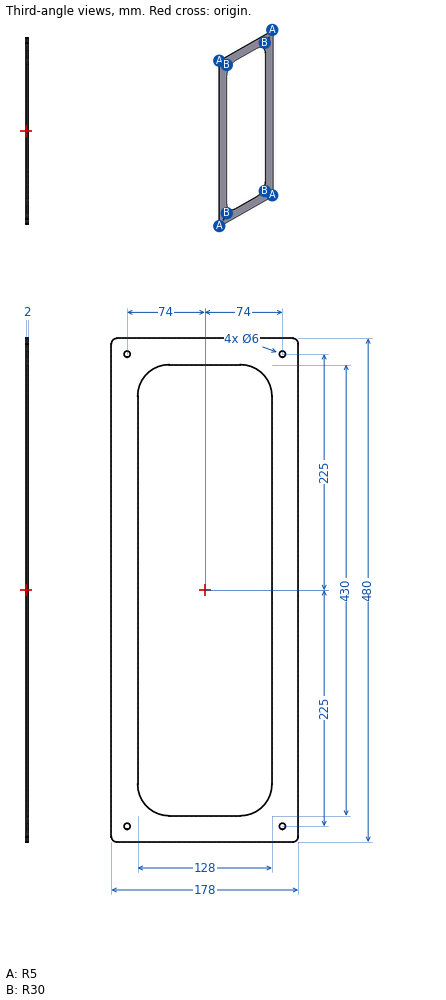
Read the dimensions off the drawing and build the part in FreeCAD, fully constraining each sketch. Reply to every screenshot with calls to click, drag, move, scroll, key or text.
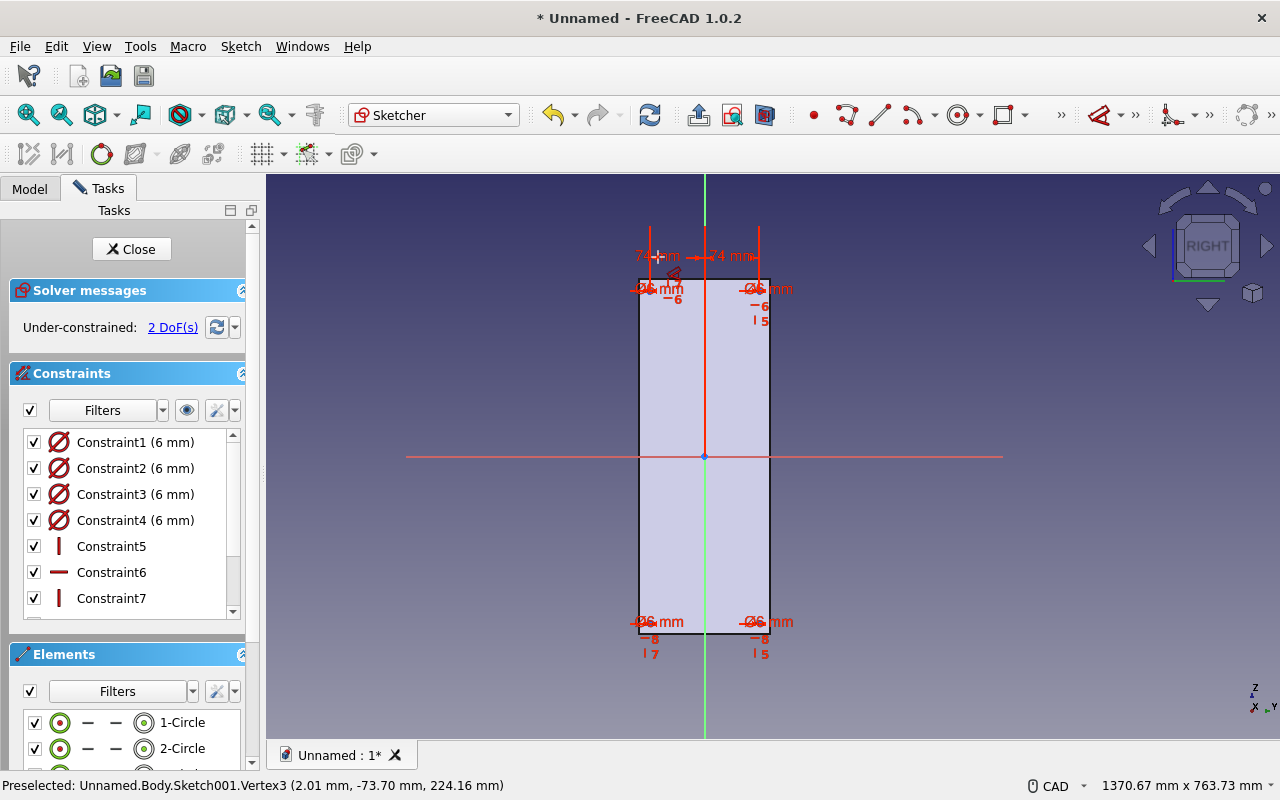
click(759, 291)
click(793, 374)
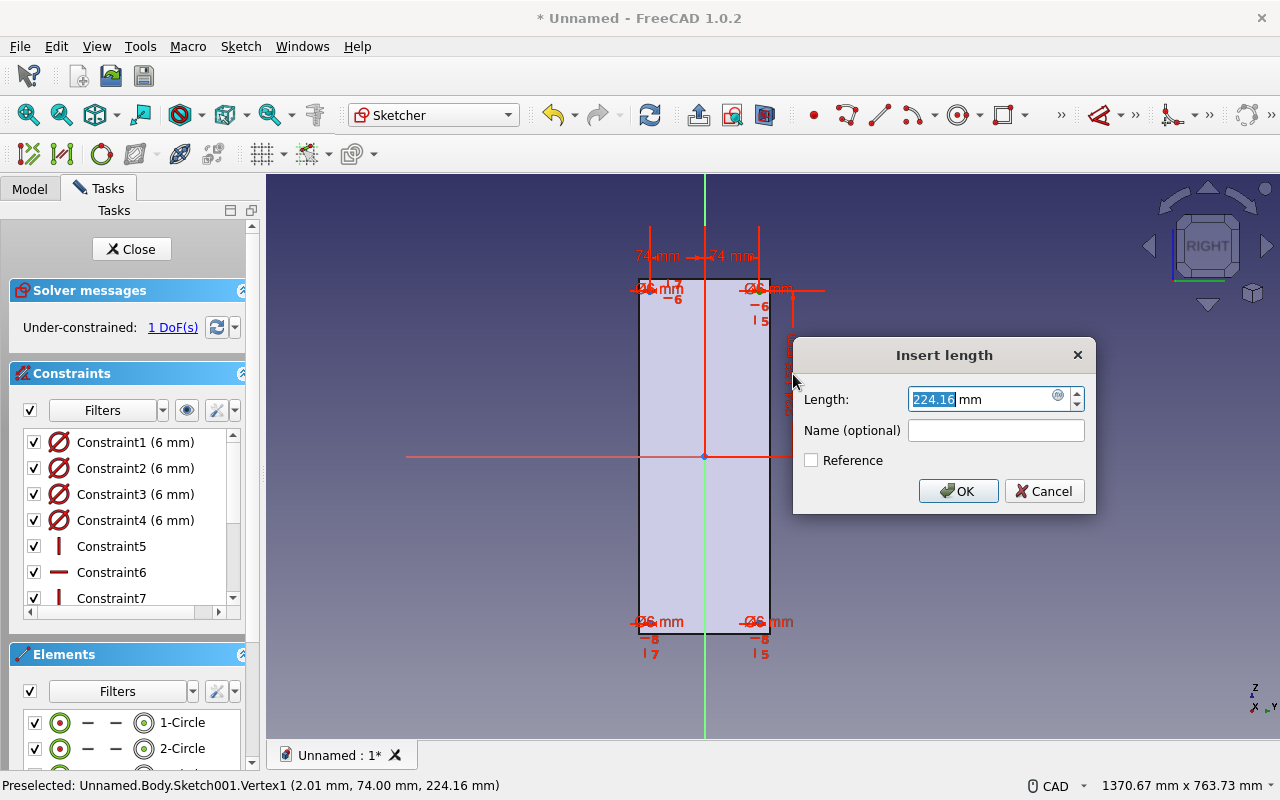
text(225)
key(Return)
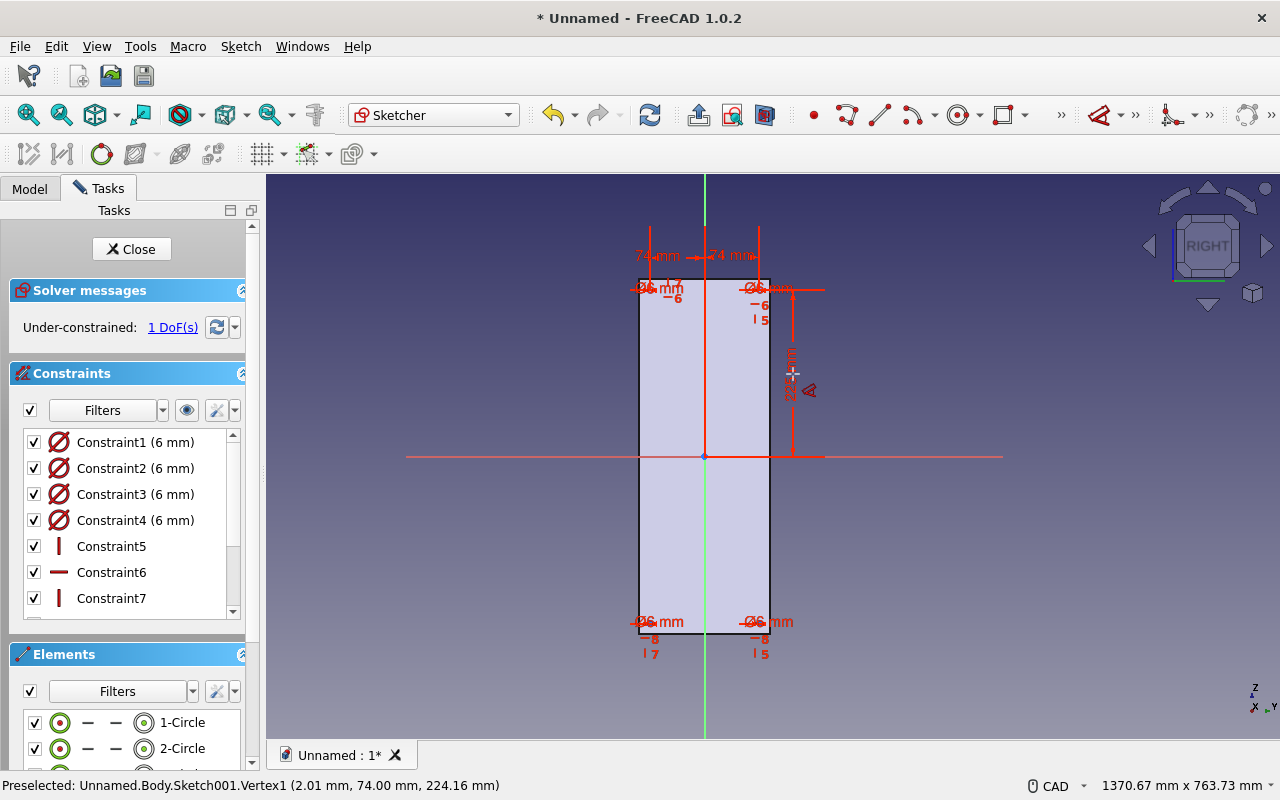
click(759, 624)
click(793, 540)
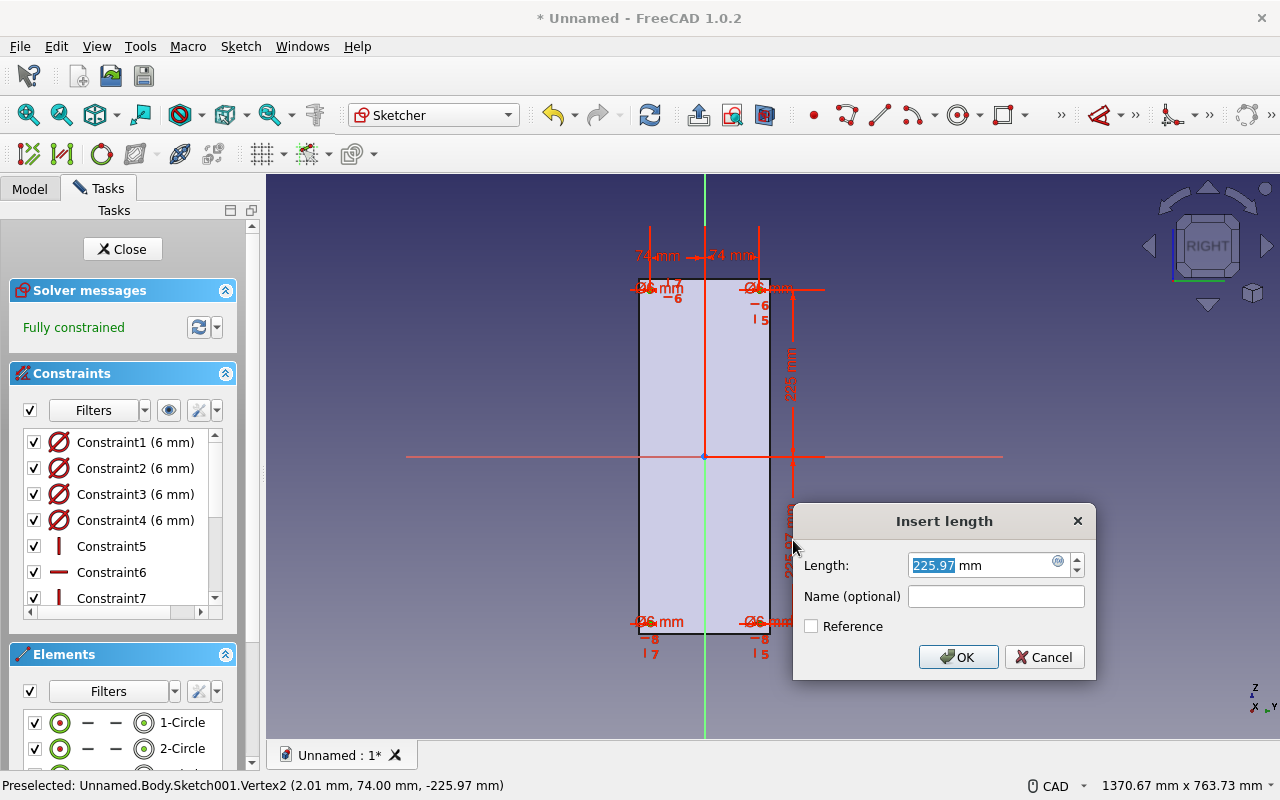
text(225)
key(Return)
key(Escape)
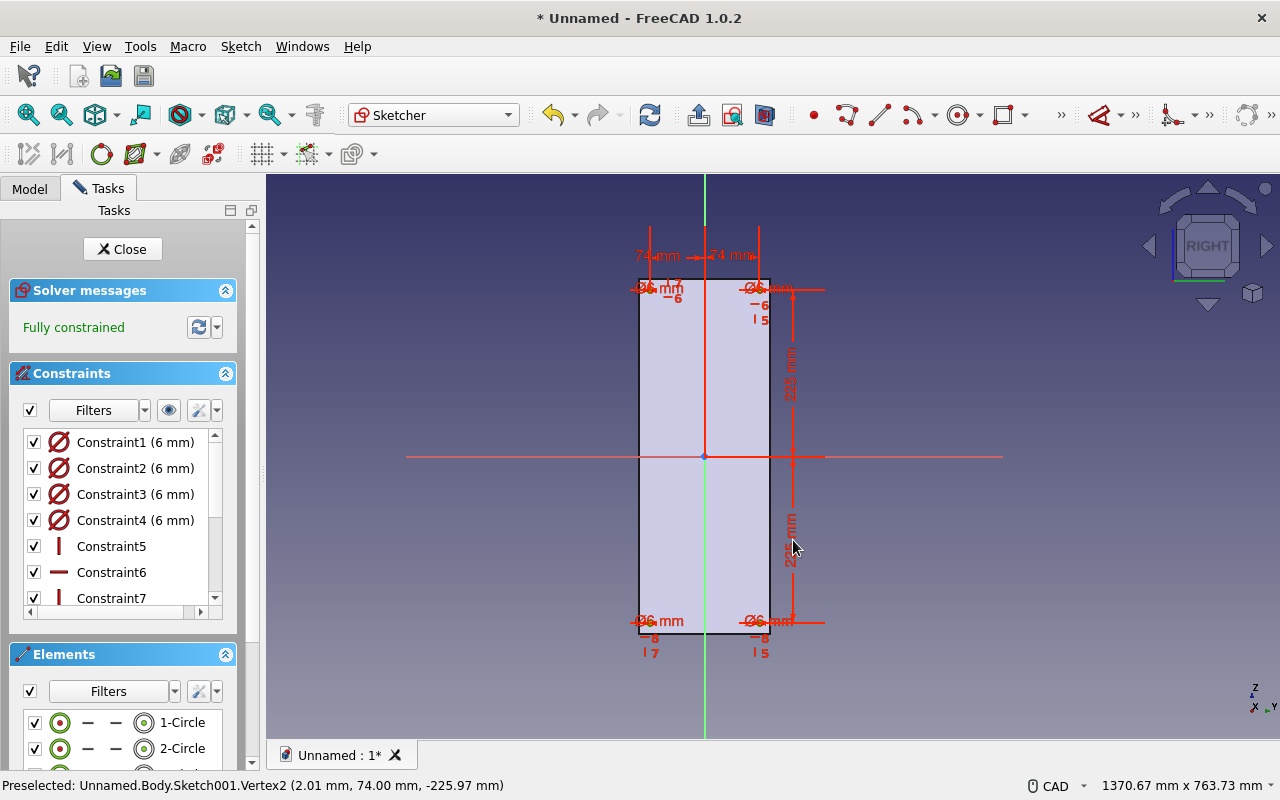
click(123, 249)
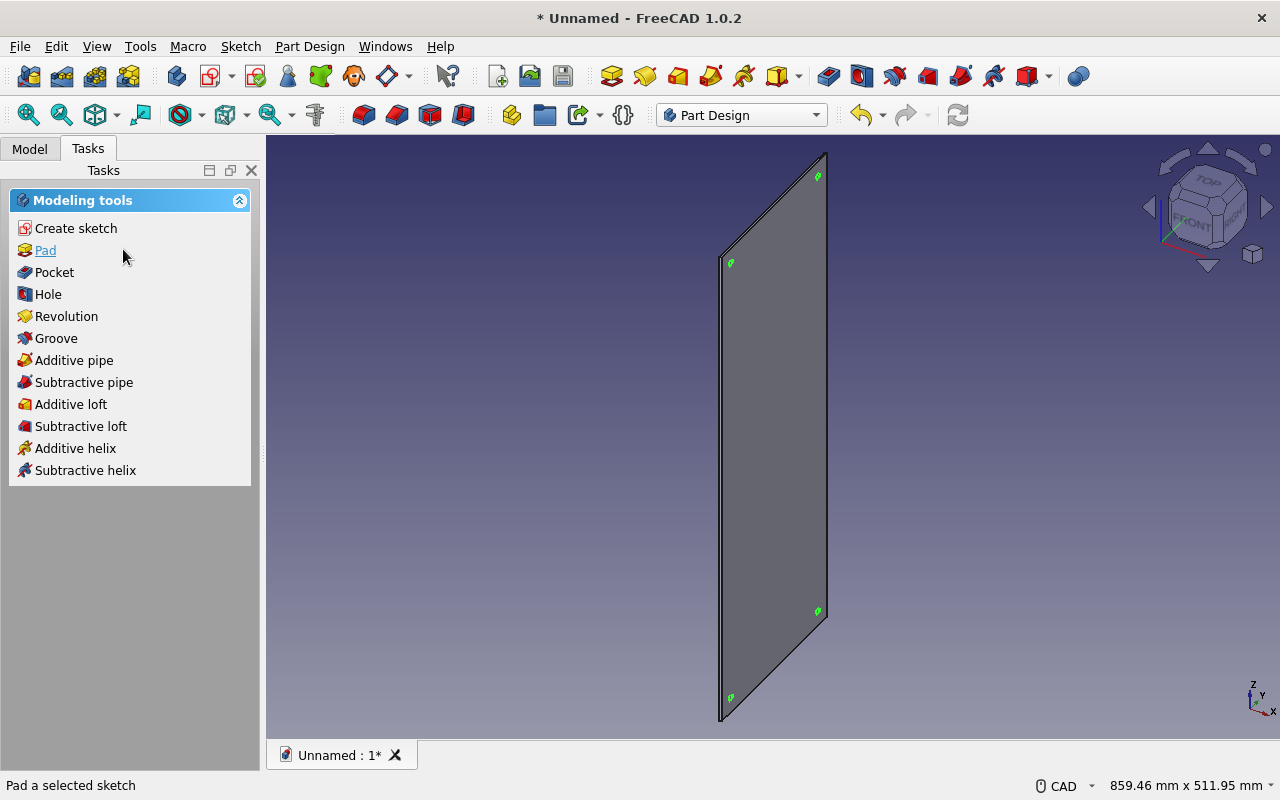
click(829, 76)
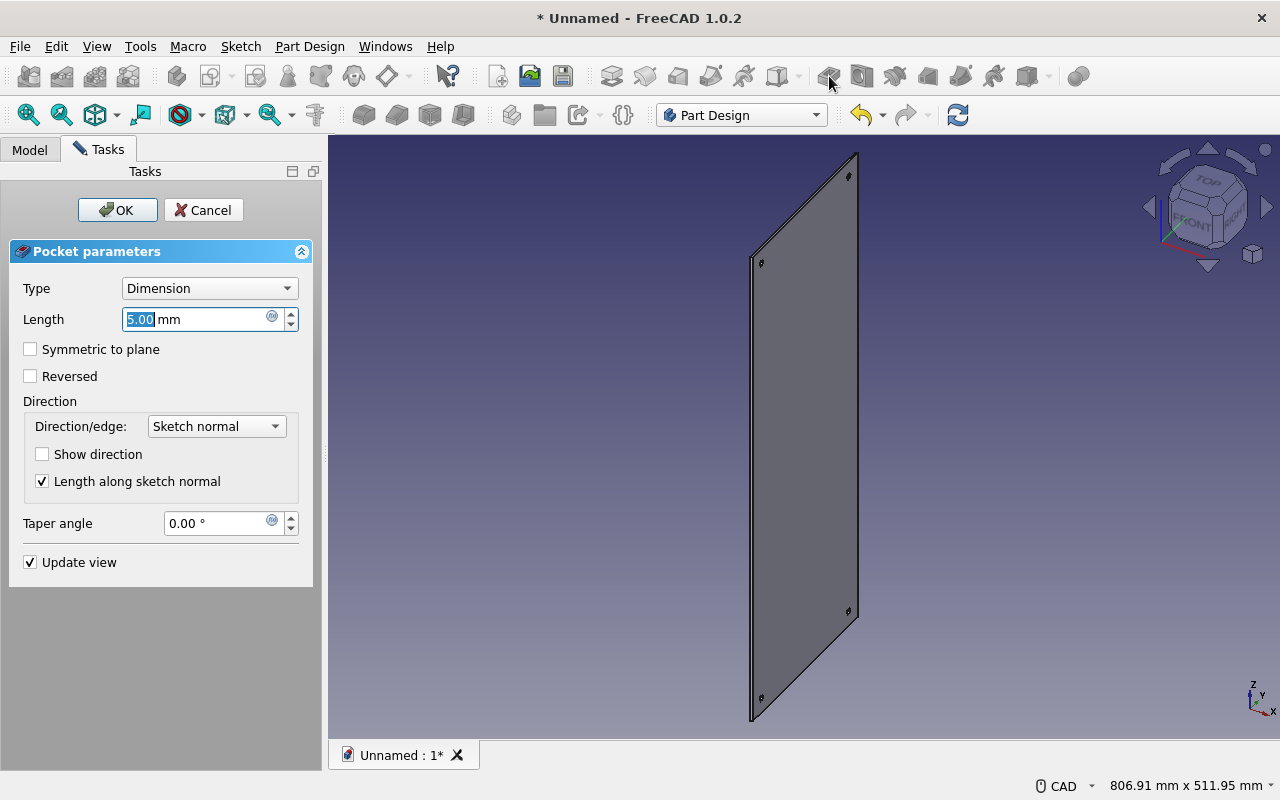
click(210, 288)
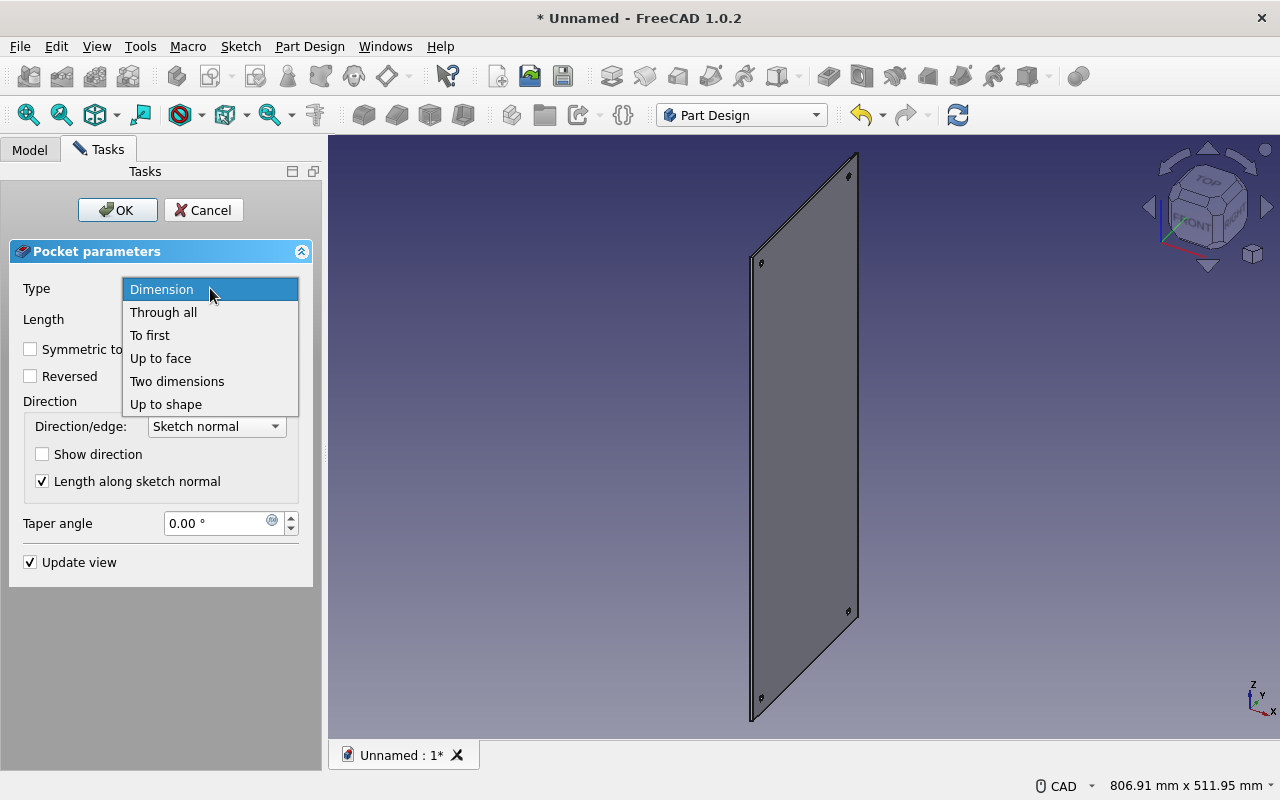
click(208, 312)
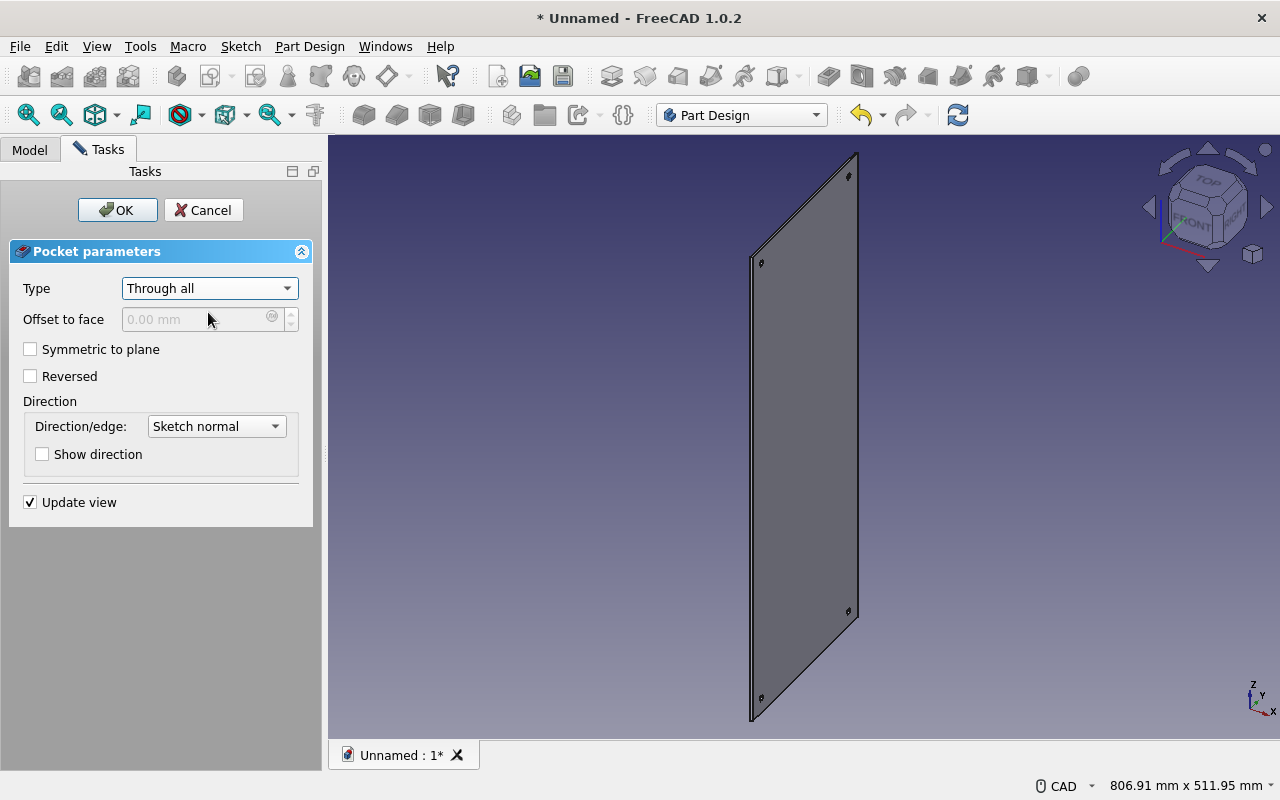
click(118, 210)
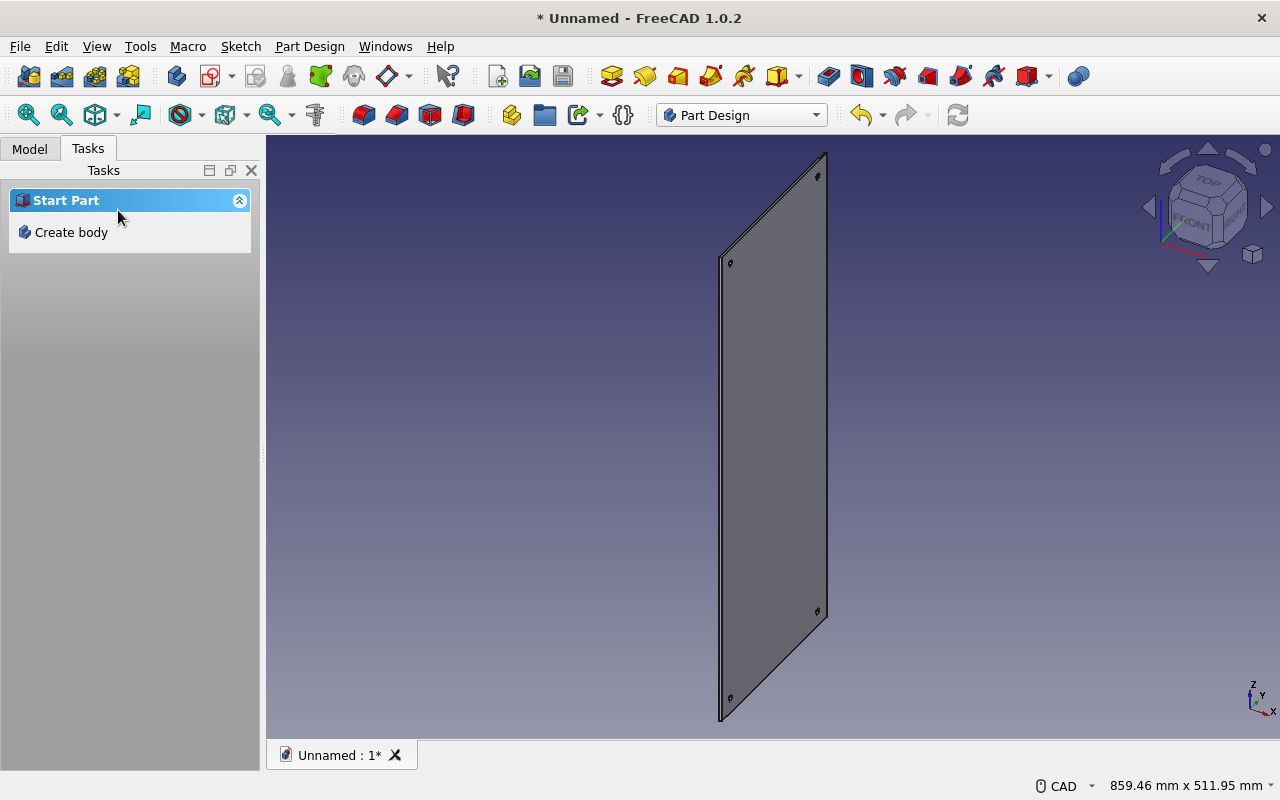
key(0)